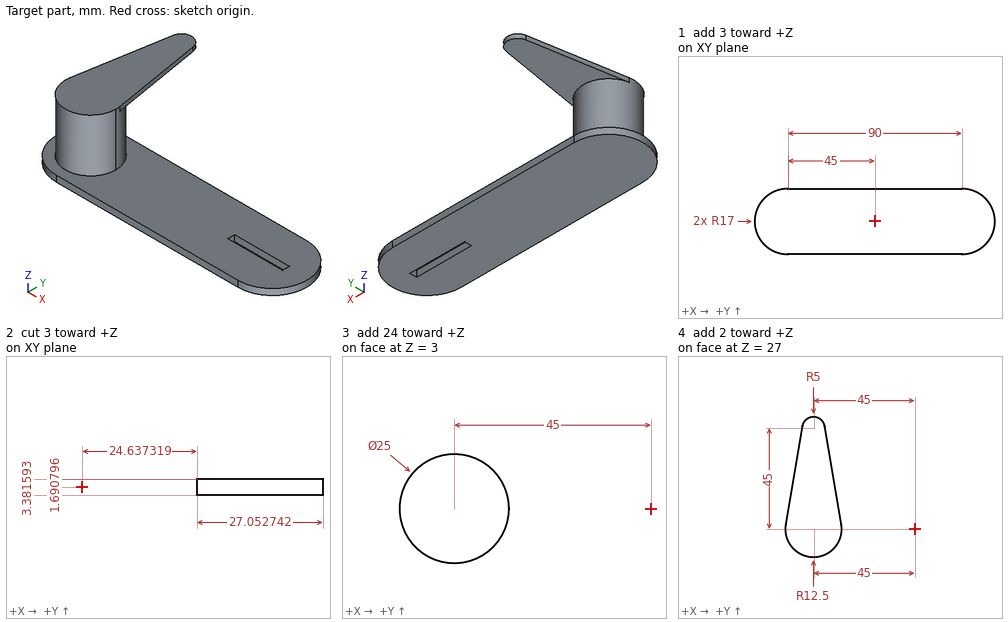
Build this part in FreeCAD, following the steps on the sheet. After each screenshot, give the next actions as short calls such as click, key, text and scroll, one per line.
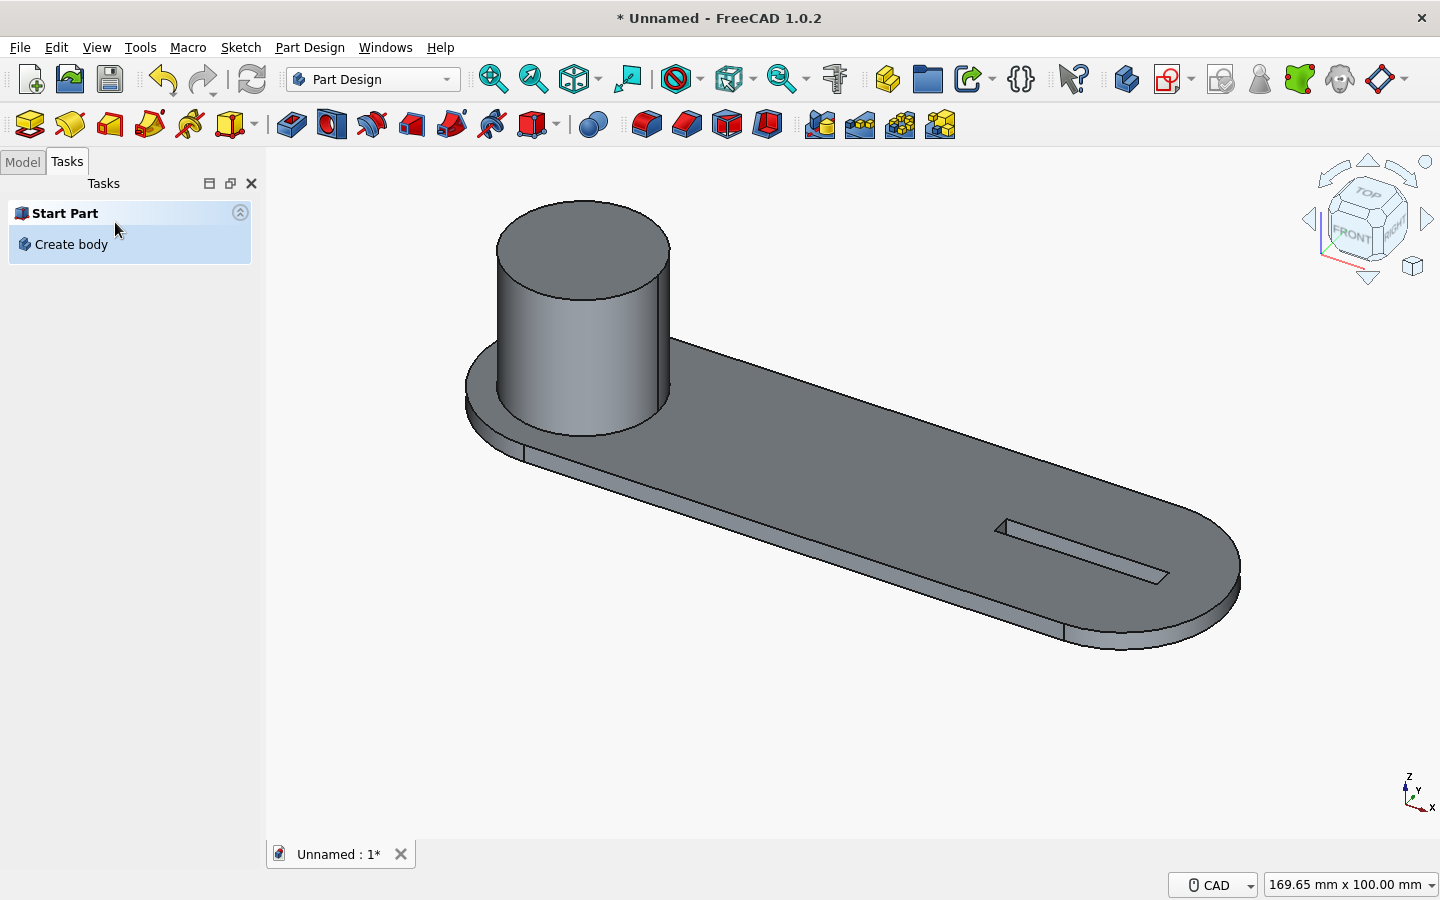
click(583, 250)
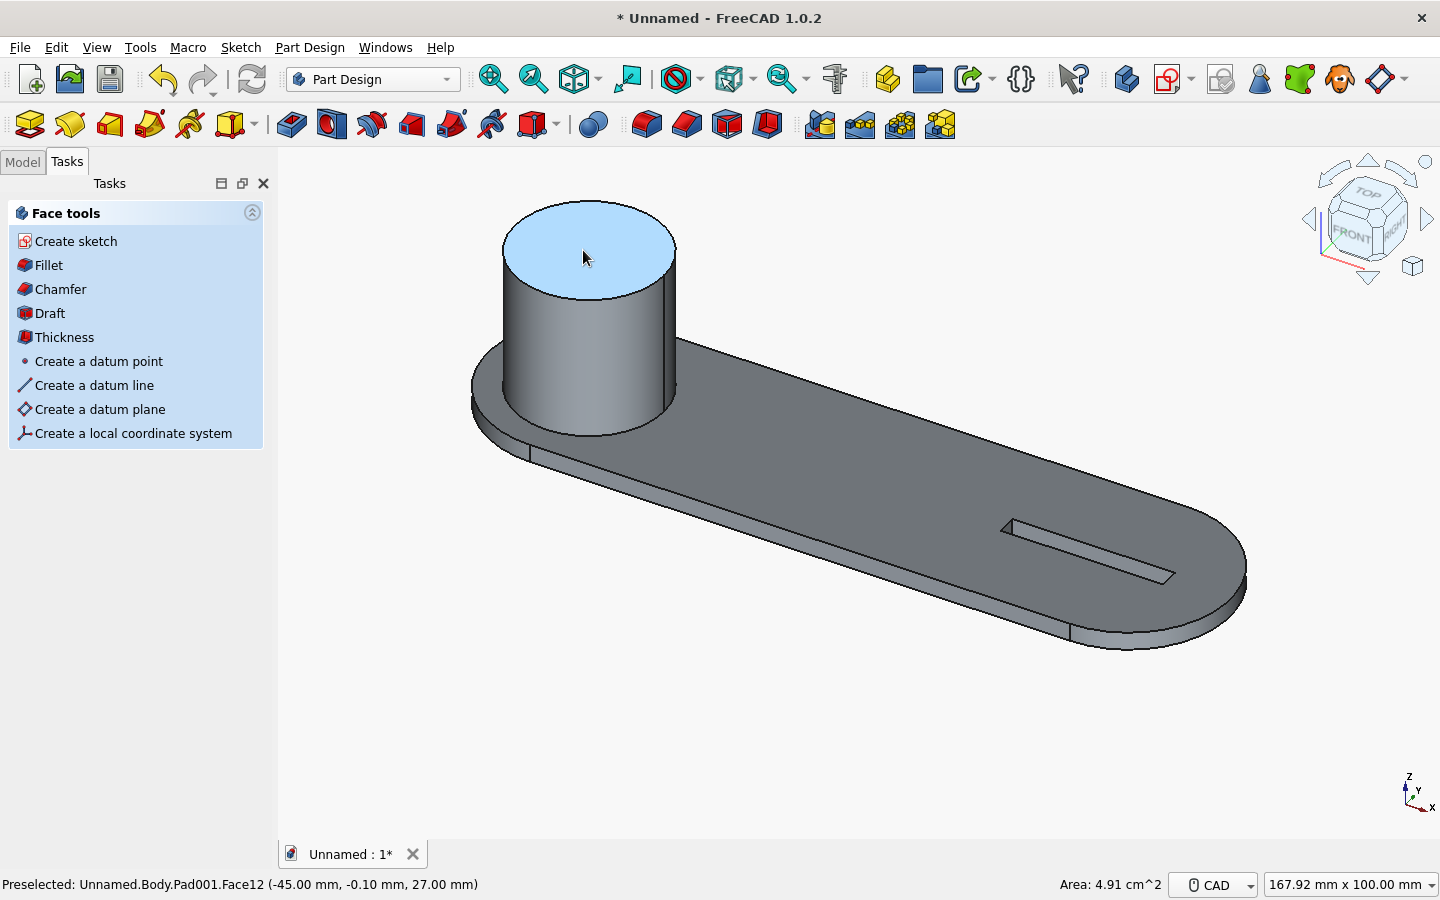
click(1168, 80)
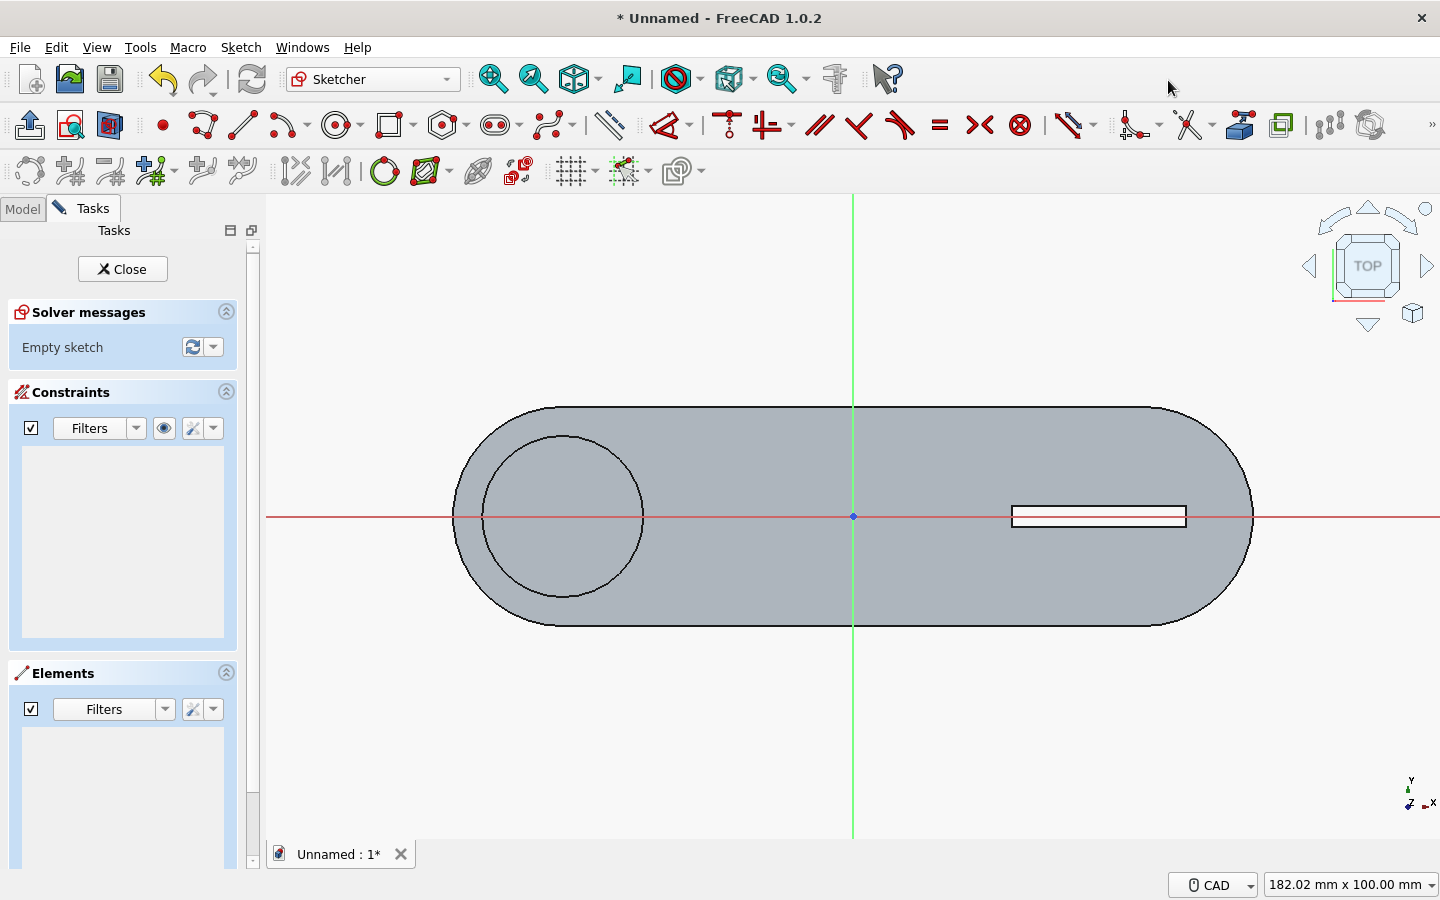
scroll(1275, 811, down, 1)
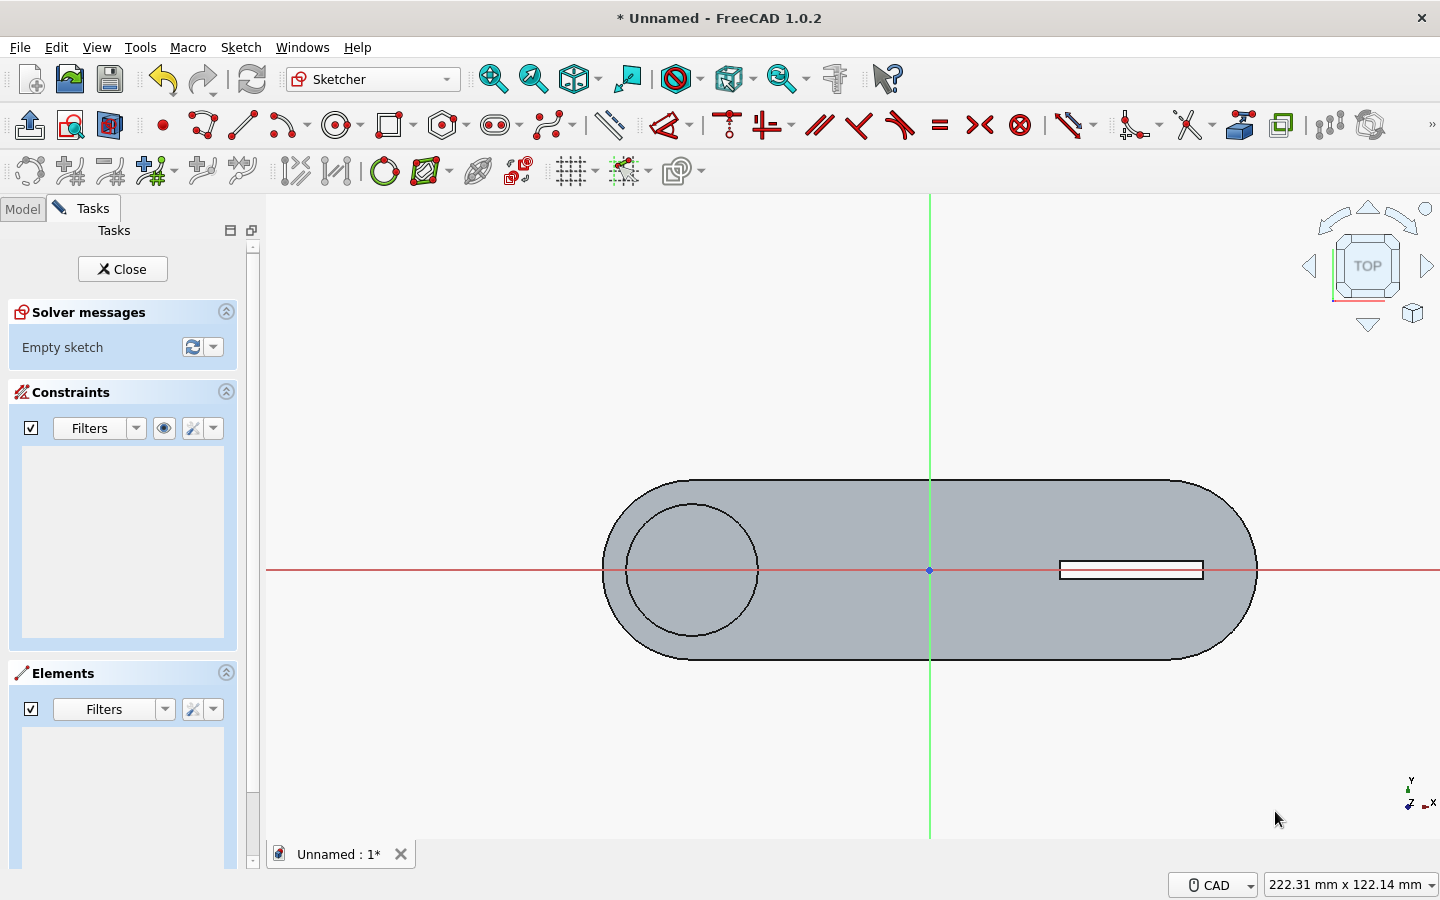
click(244, 126)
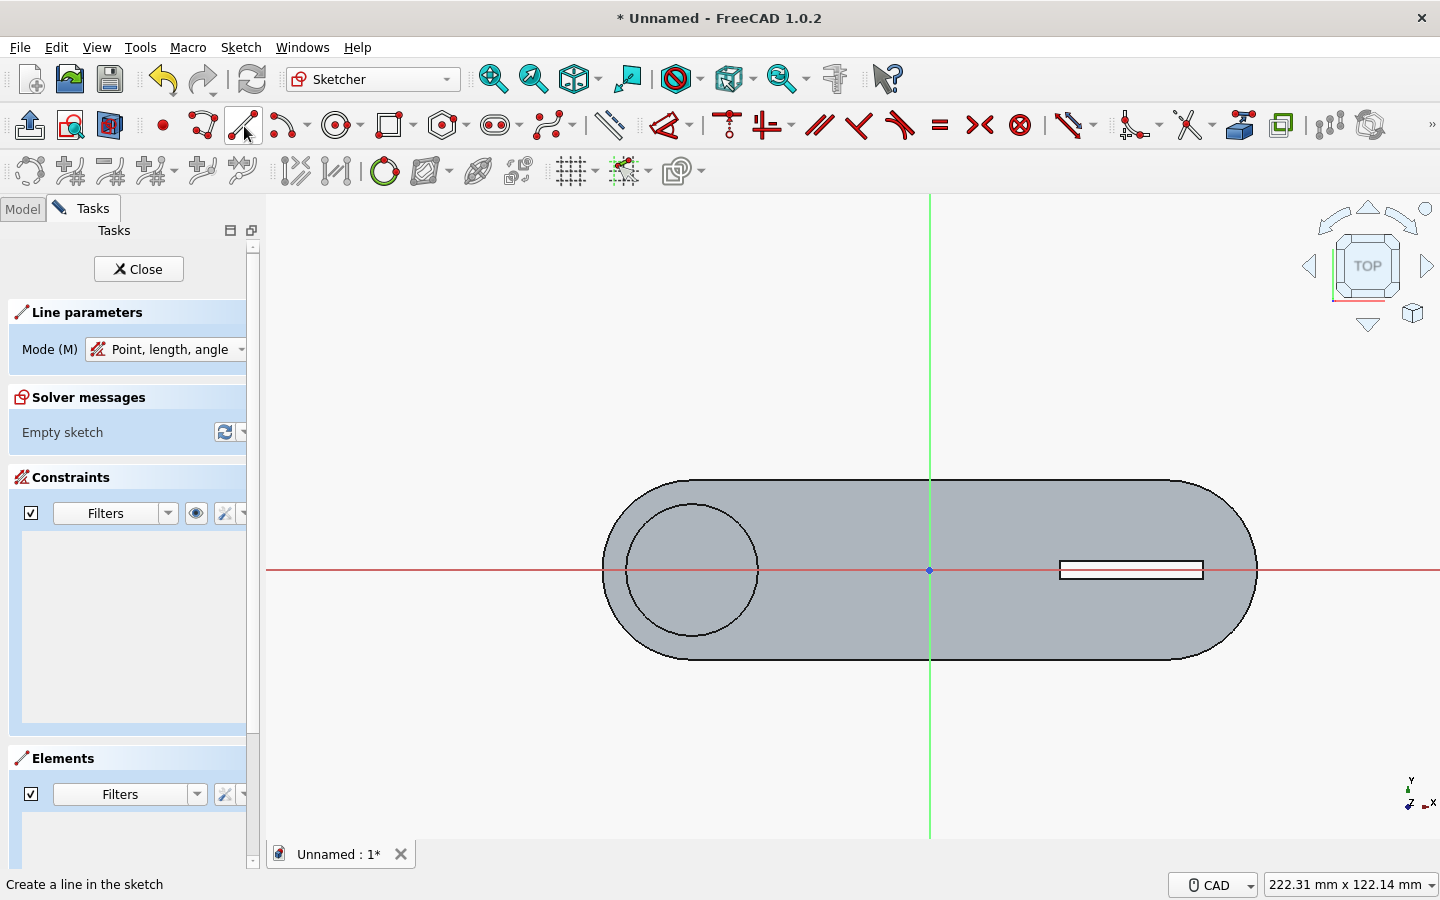
click(666, 328)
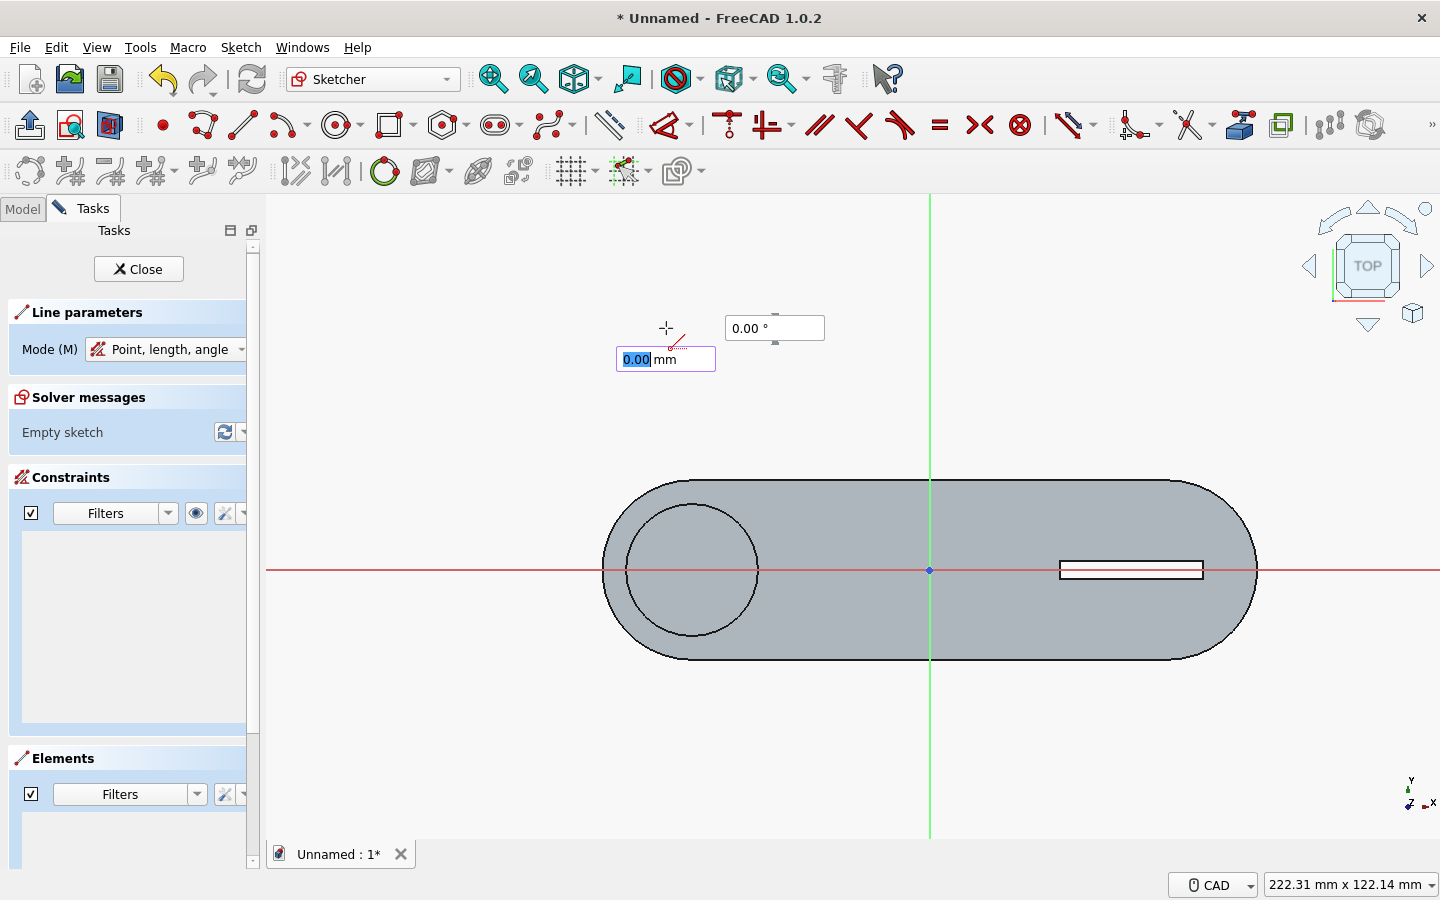
scroll(627, 559, up, 2)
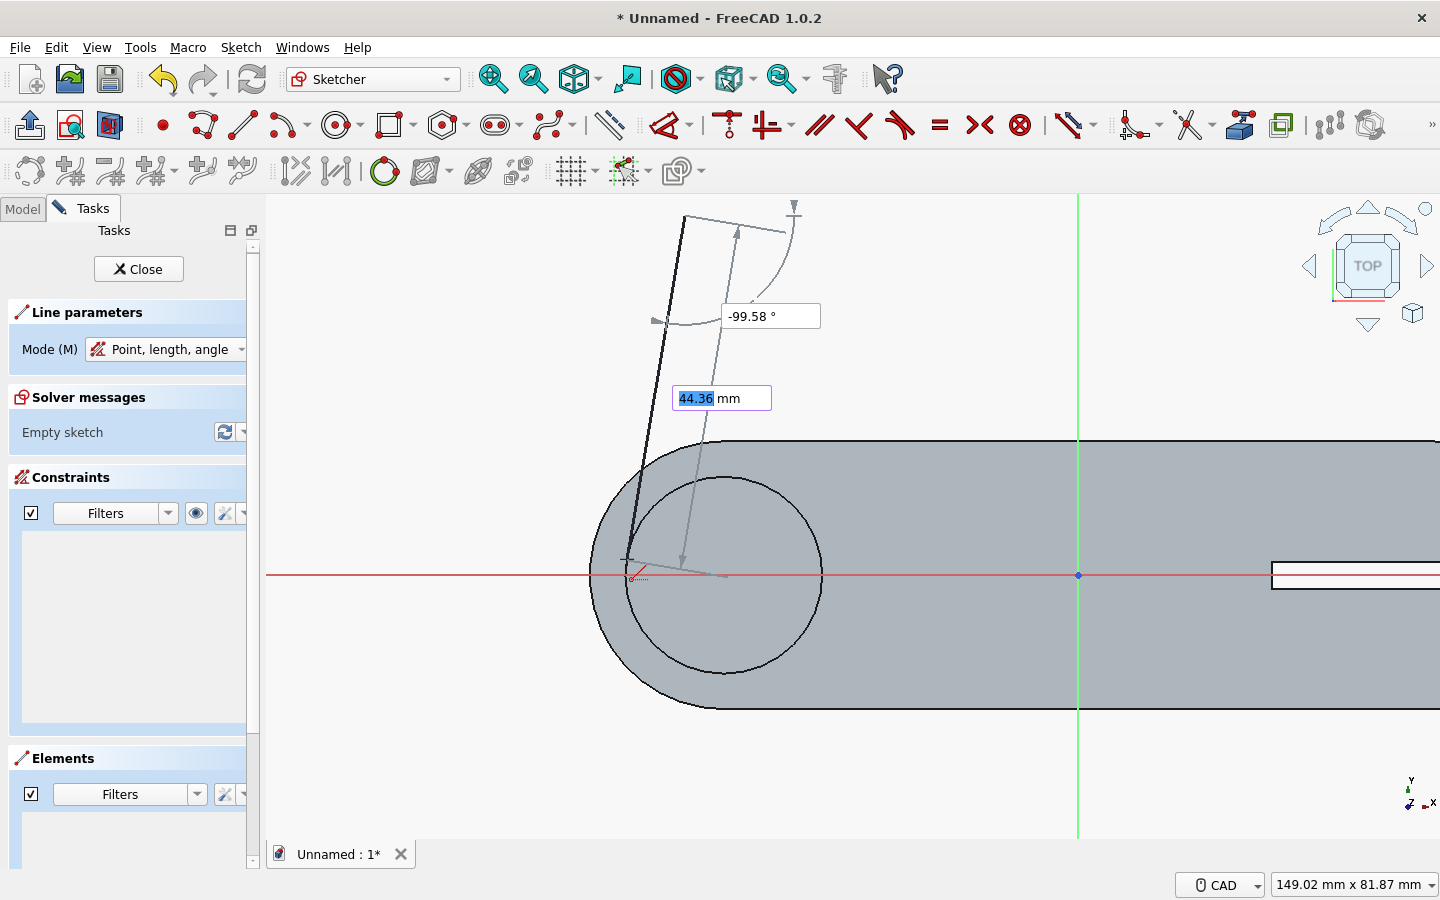
click(627, 559)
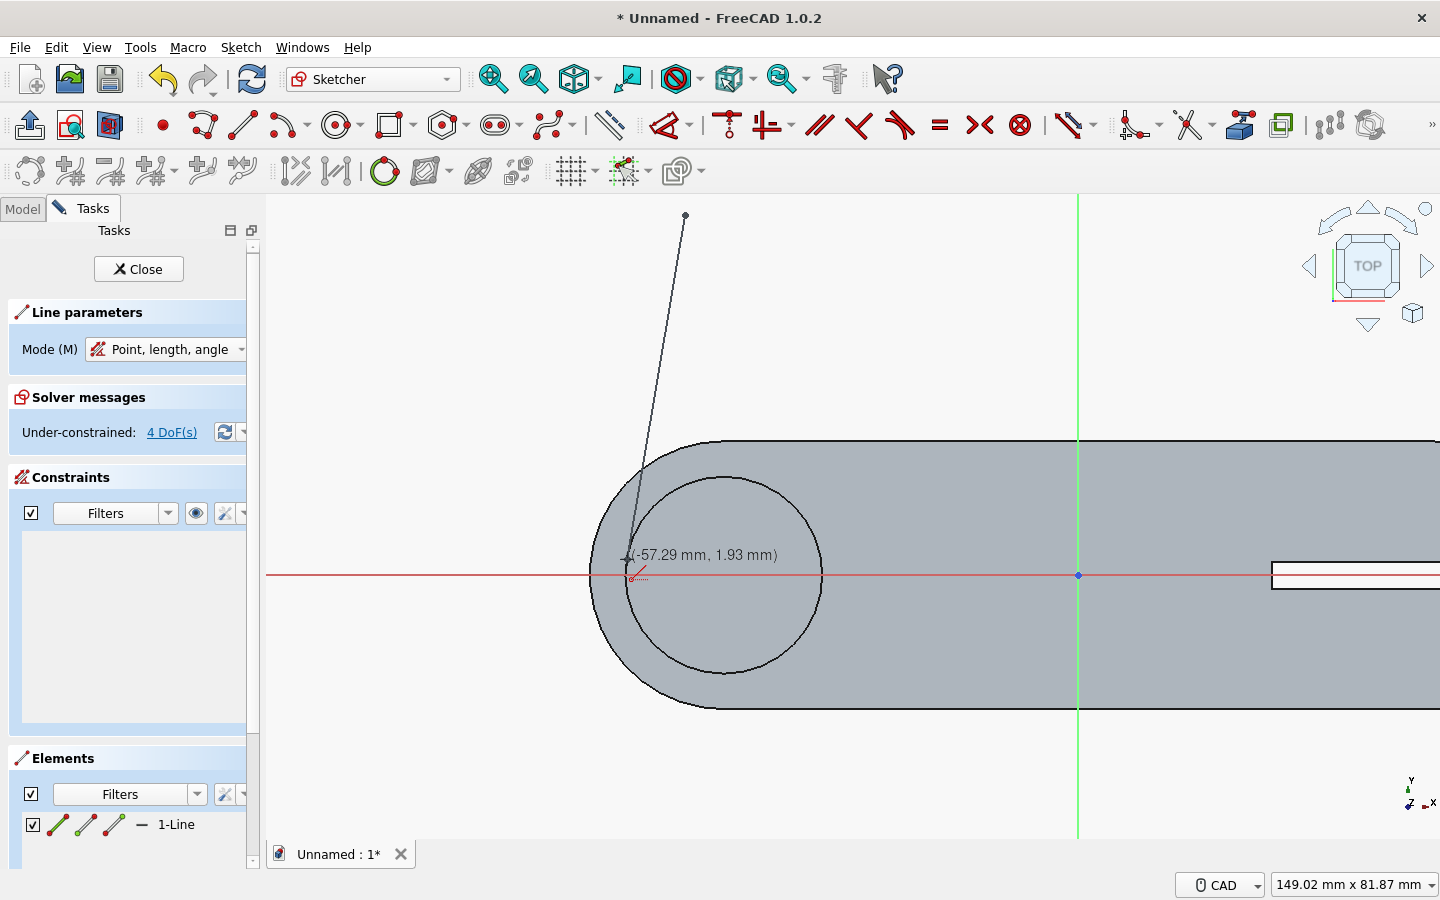
click(821, 559)